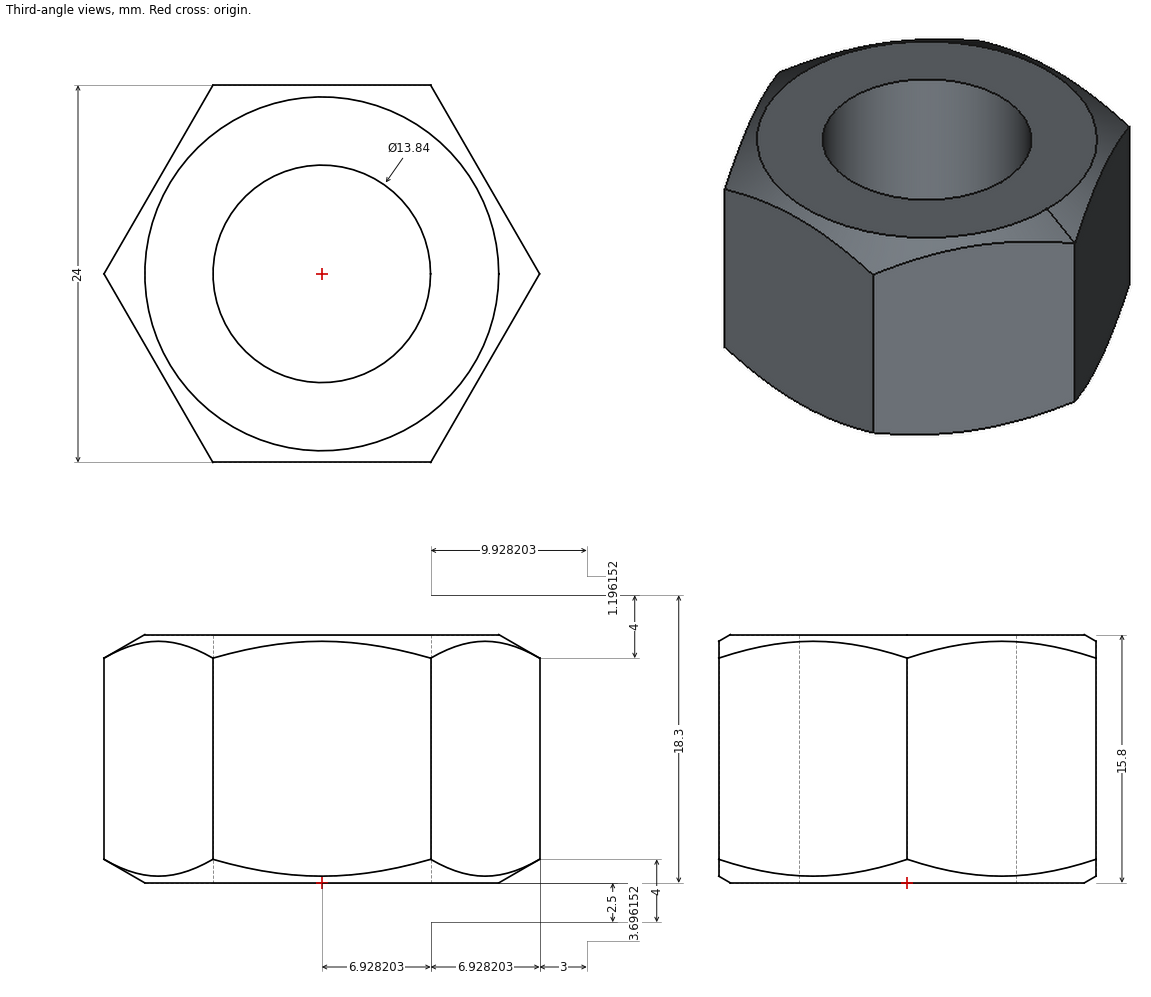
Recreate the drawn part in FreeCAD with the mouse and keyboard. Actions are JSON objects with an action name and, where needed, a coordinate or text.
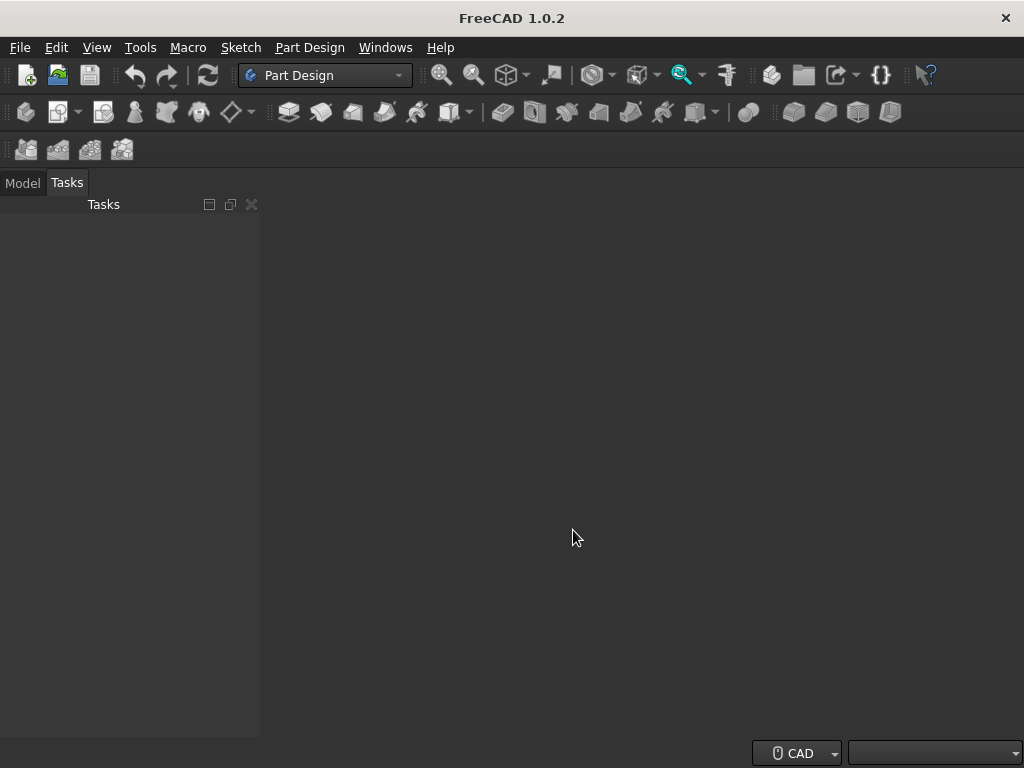
{"action": "left_click", "coordinate": [26, 76]}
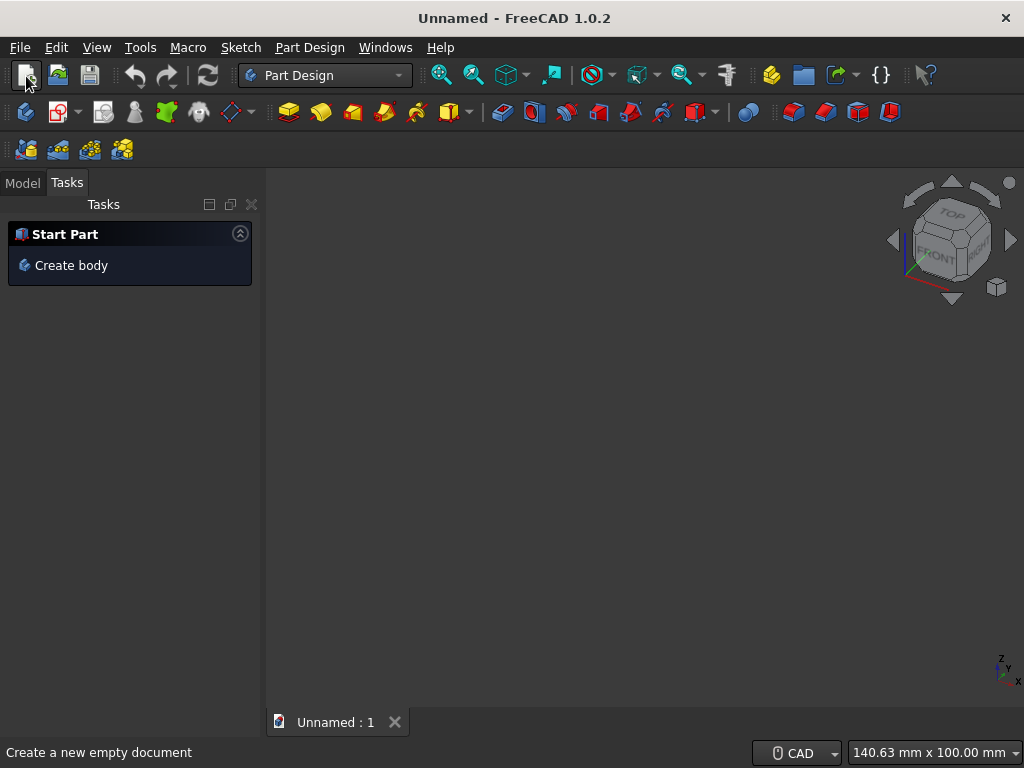
{"action": "left_click", "coordinate": [58, 112]}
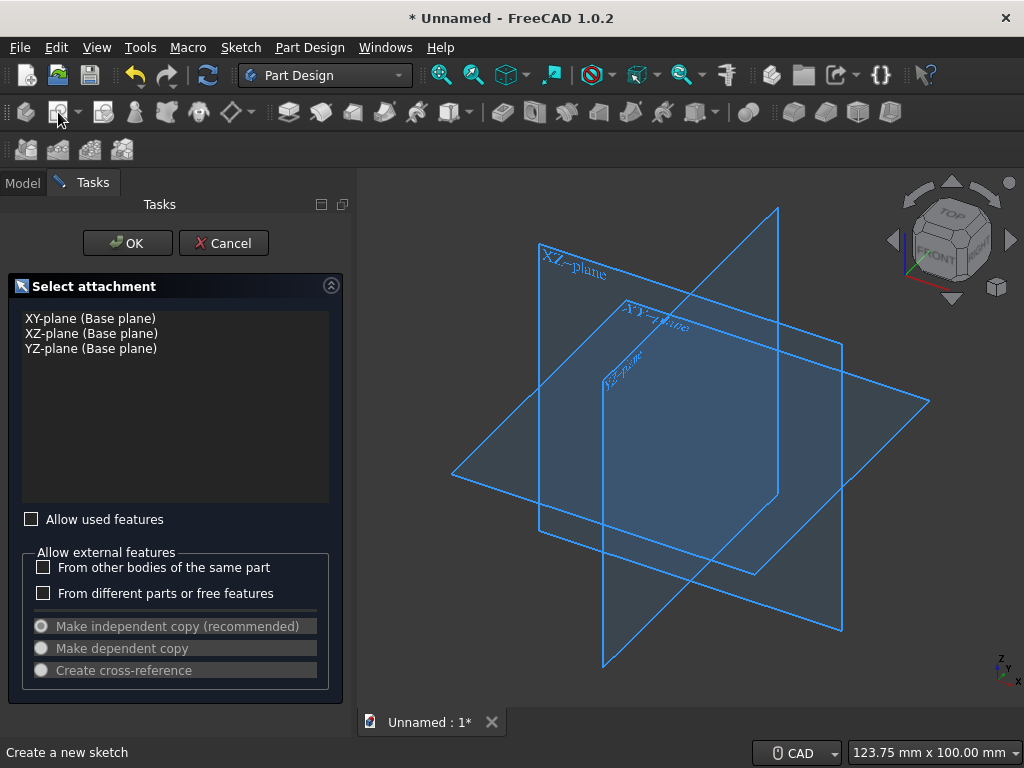
{"action": "left_click", "coordinate": [82, 318]}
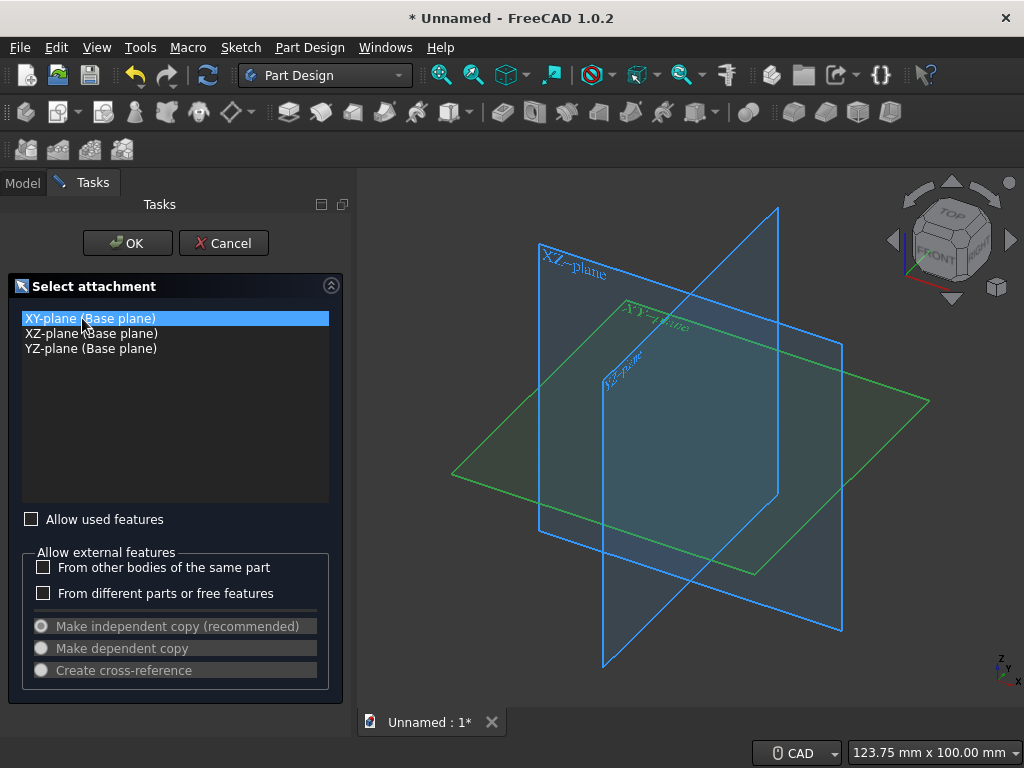
{"action": "left_click", "coordinate": [128, 243]}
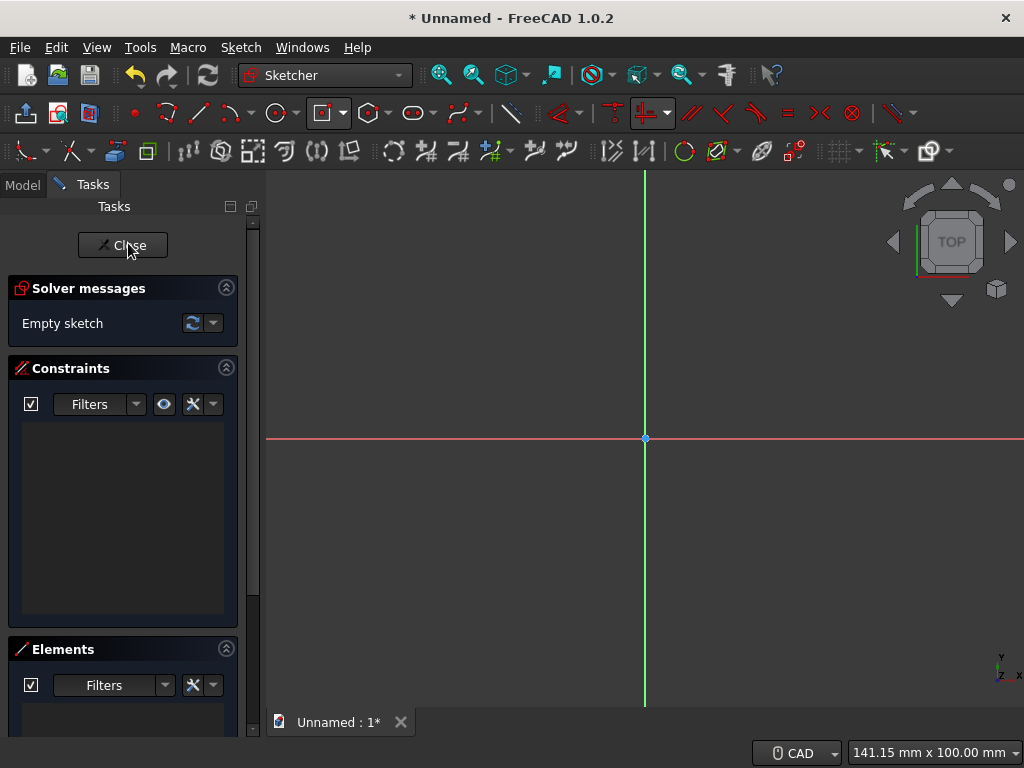
{"action": "scroll", "coordinate": [685, 439], "scroll_direction": "up", "scroll_amount": 5}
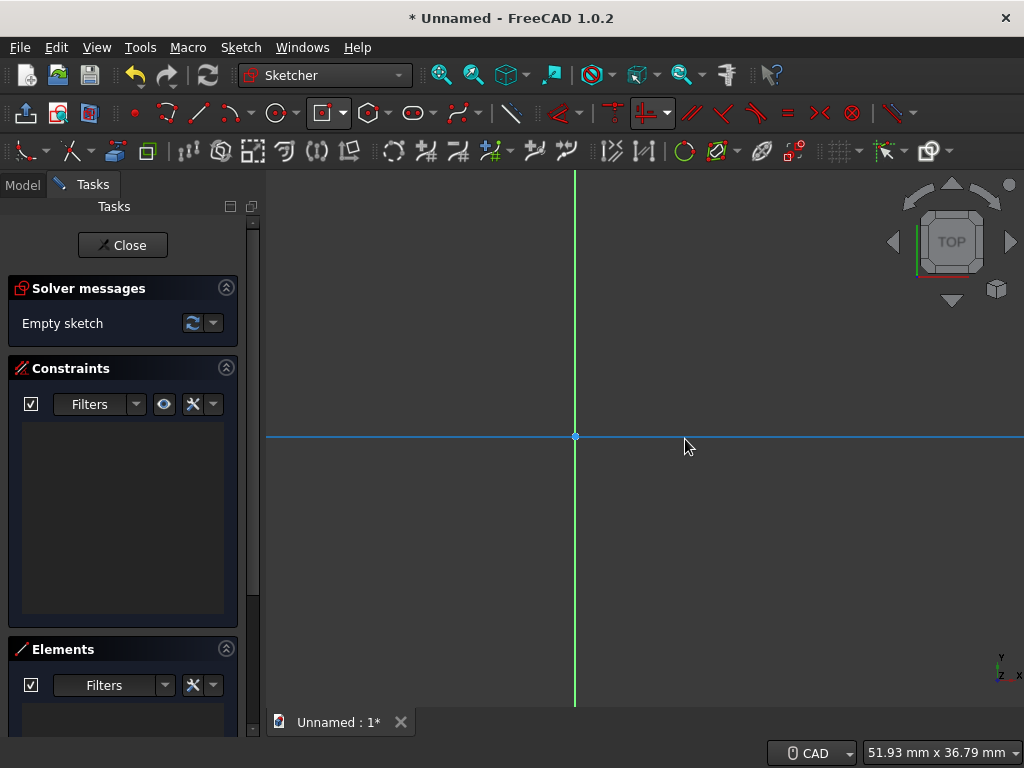
{"action": "left_click", "coordinate": [368, 114]}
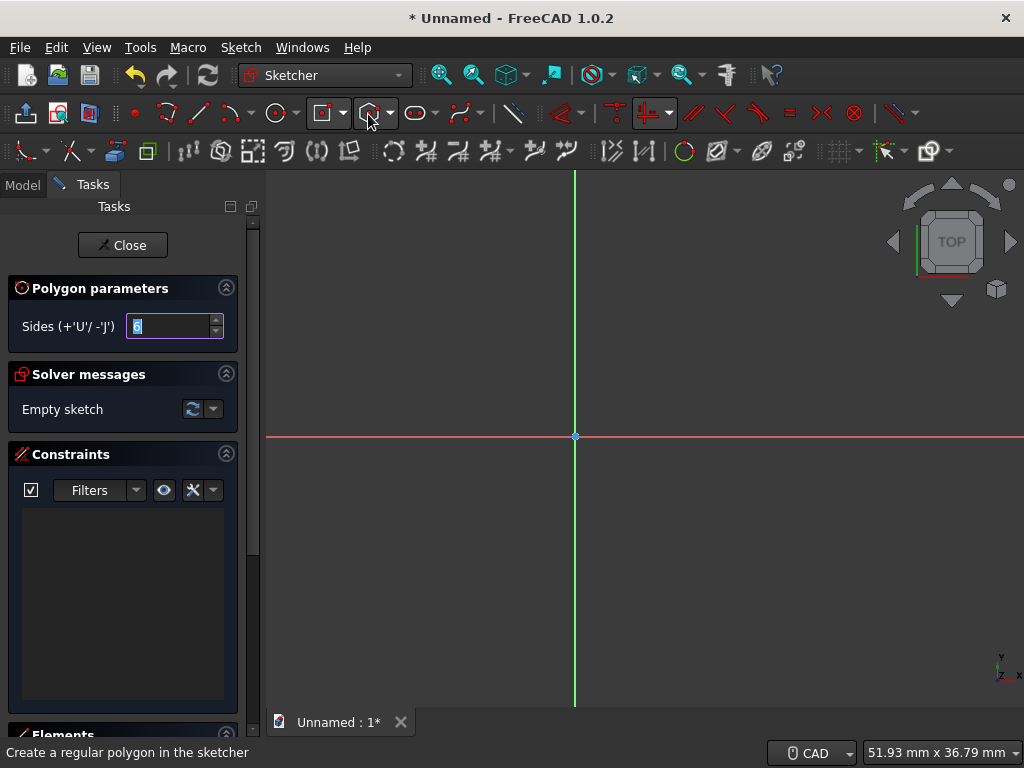
{"action": "left_click", "coordinate": [575, 437]}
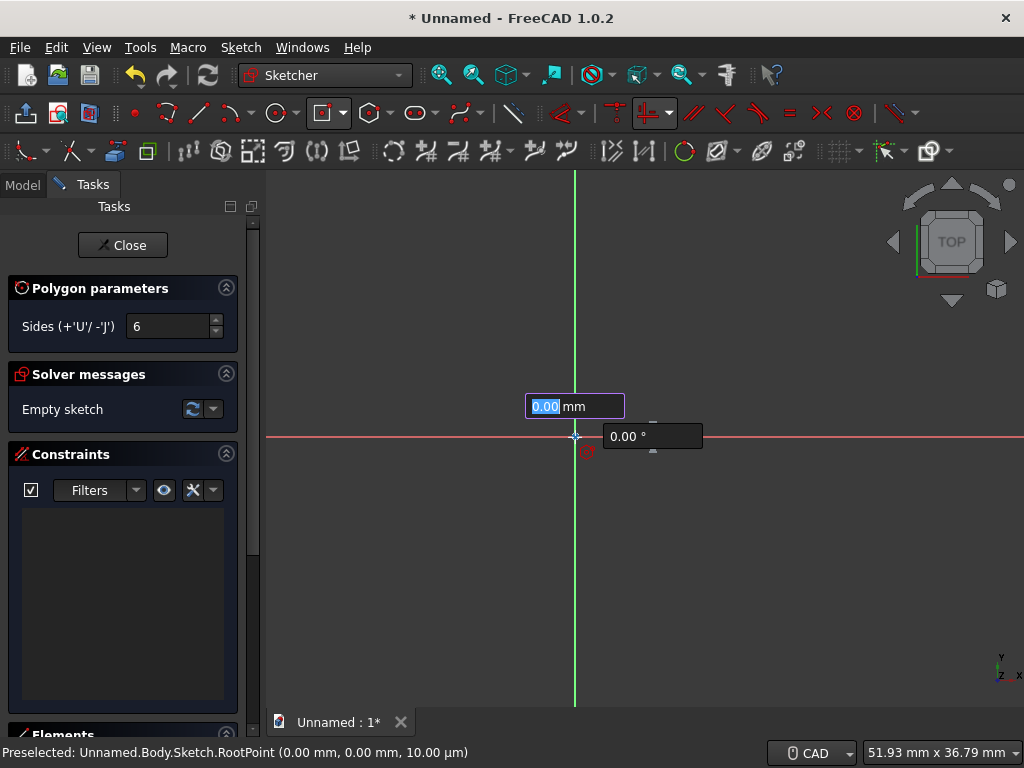
{"action": "left_click", "coordinate": [778, 437]}
{"action": "key", "text": "Escape"}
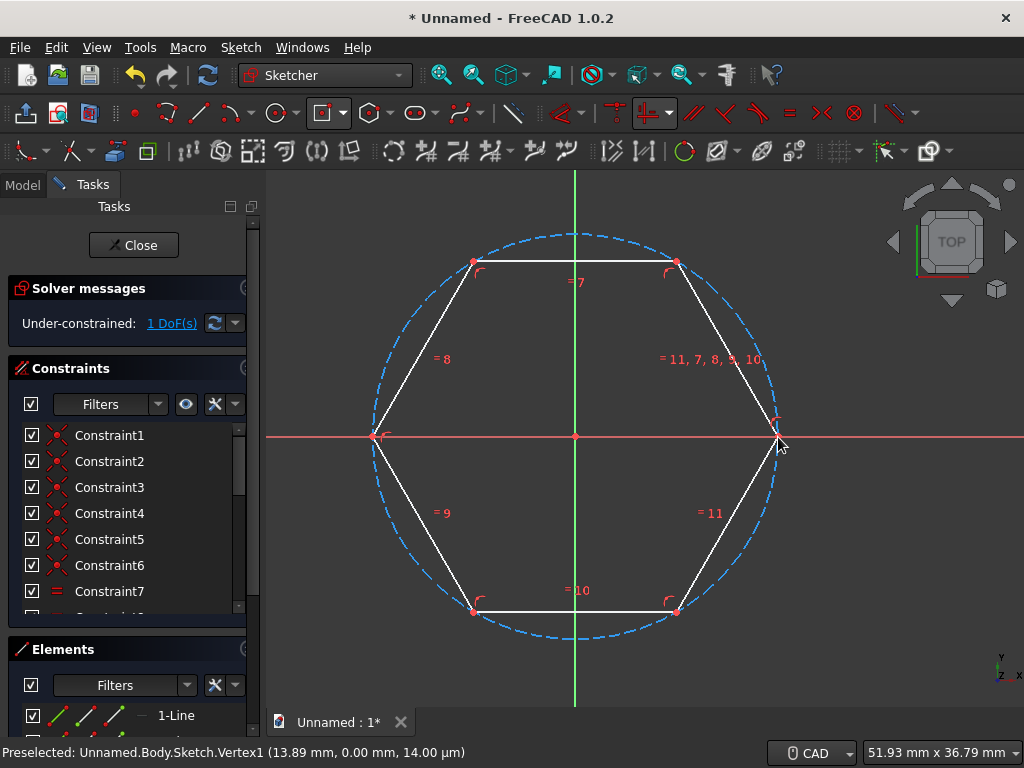
{"action": "left_click", "coordinate": [560, 114]}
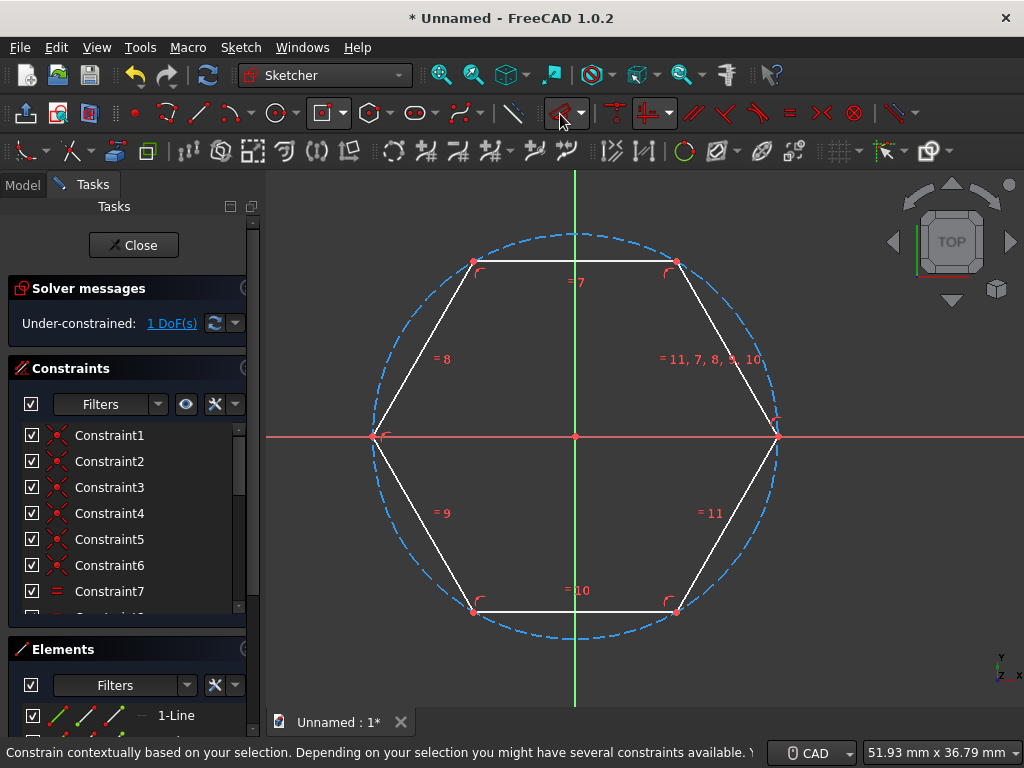
{"action": "left_click", "coordinate": [474, 612]}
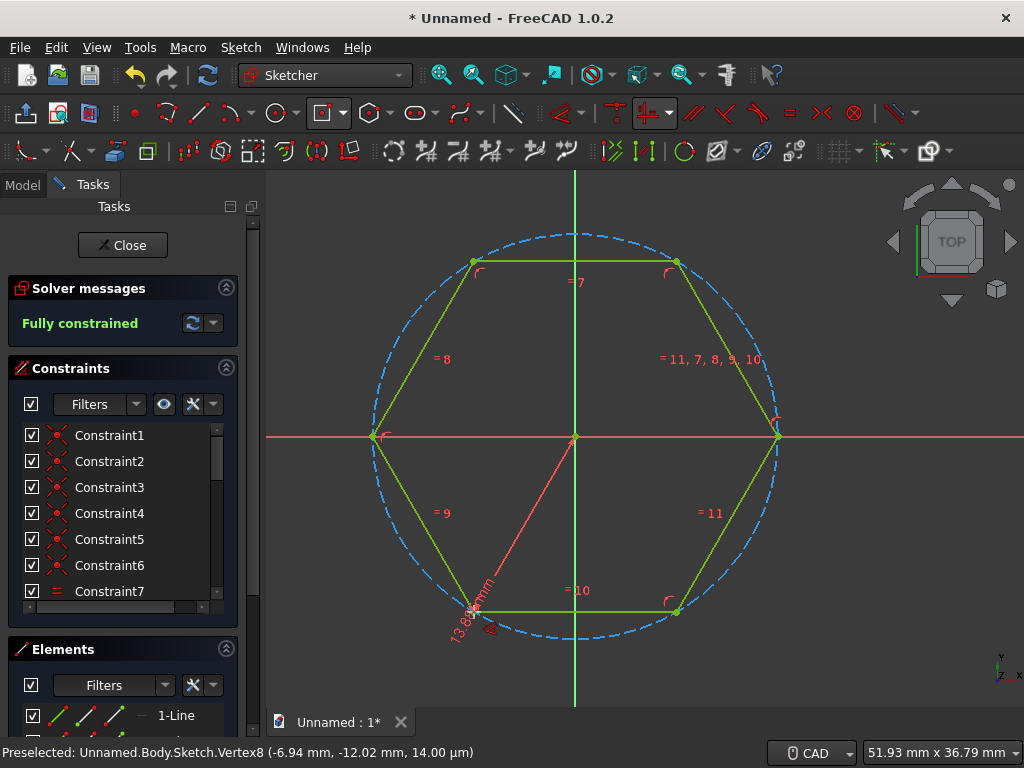
{"action": "left_click", "coordinate": [677, 261]}
{"action": "left_click", "coordinate": [711, 356]}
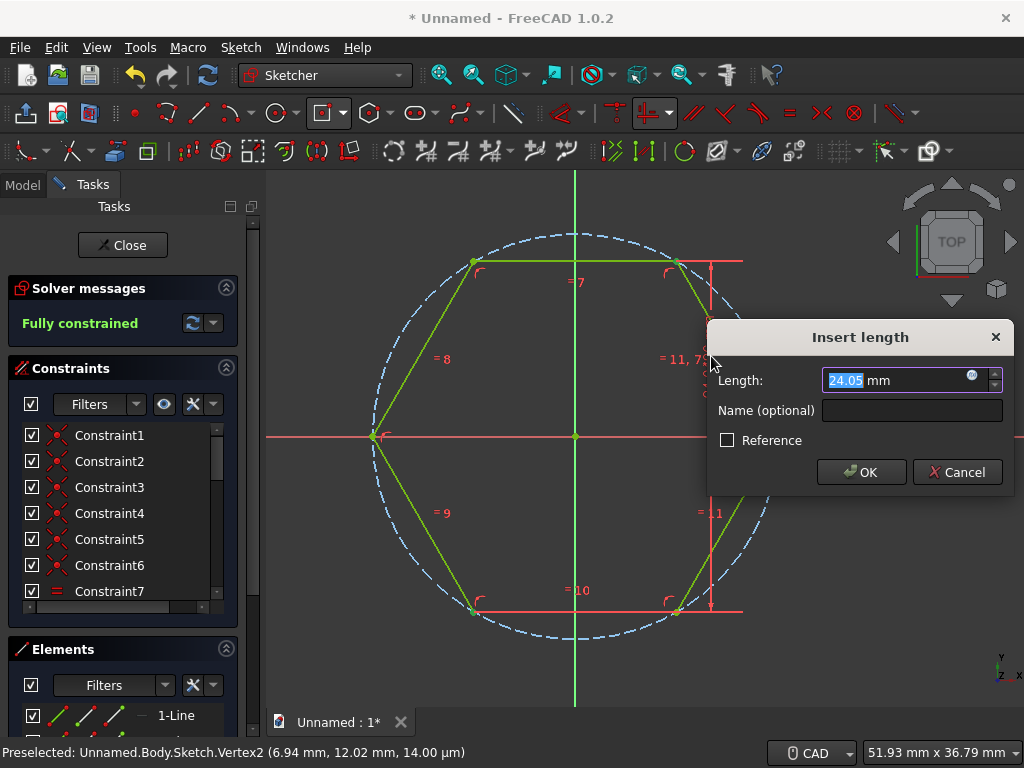
{"action": "type", "text": "24"}
{"action": "key", "text": "Return"}
{"action": "key", "text": "Escape"}